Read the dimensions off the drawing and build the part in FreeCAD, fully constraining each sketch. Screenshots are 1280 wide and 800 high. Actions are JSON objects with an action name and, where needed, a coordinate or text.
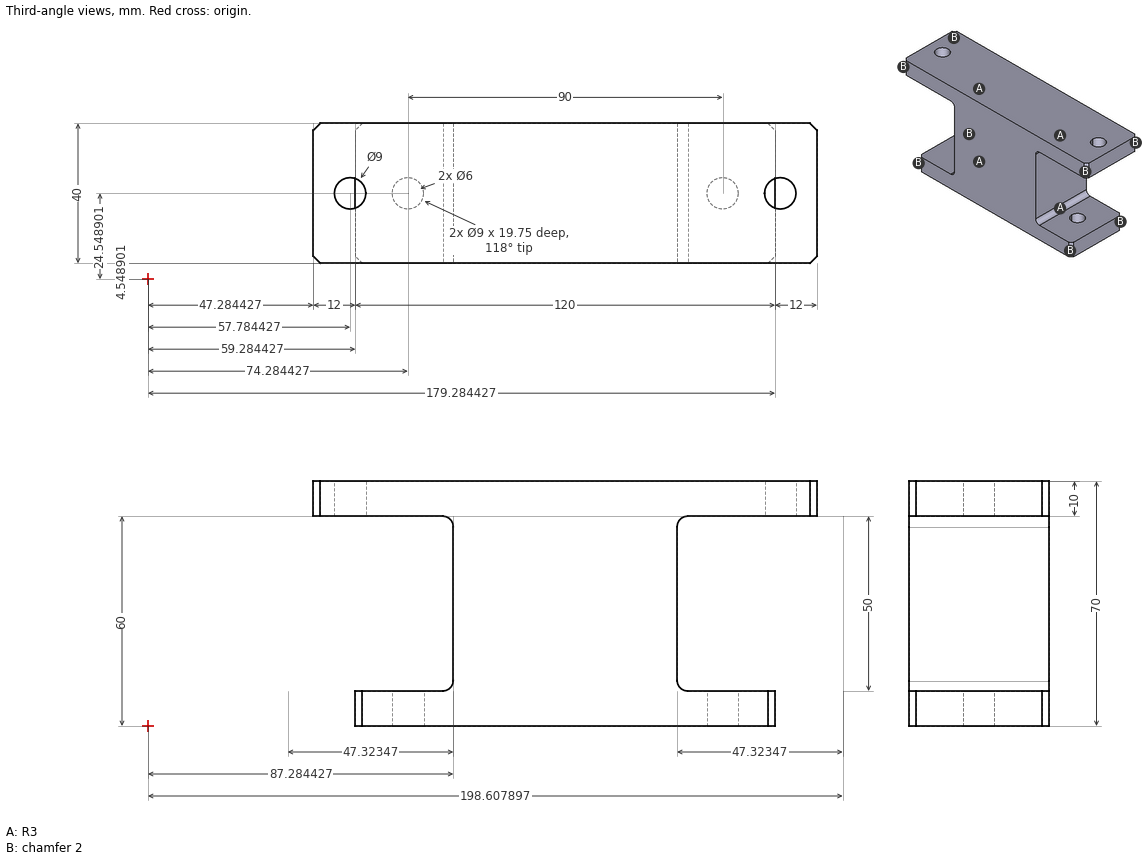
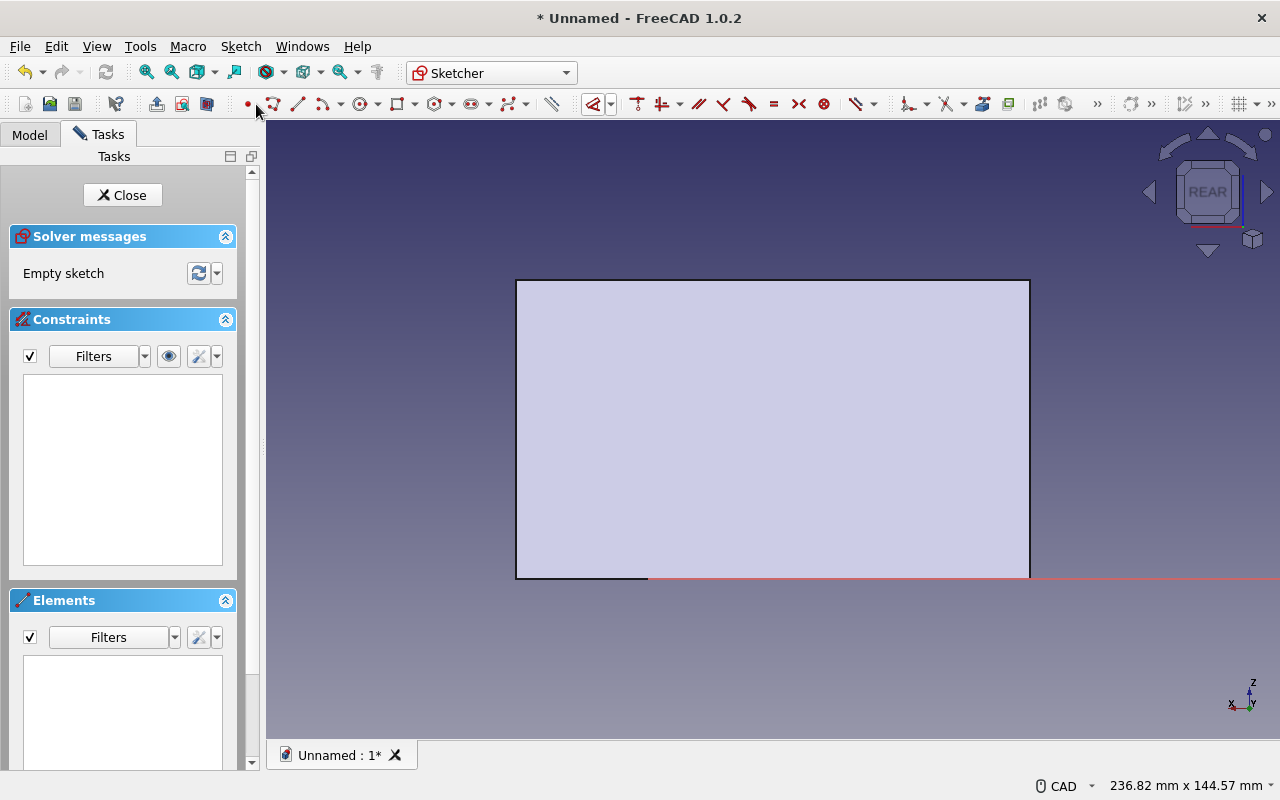
{"action": "scroll", "coordinate": [391, 386], "scroll_direction": "down", "scroll_amount": 2}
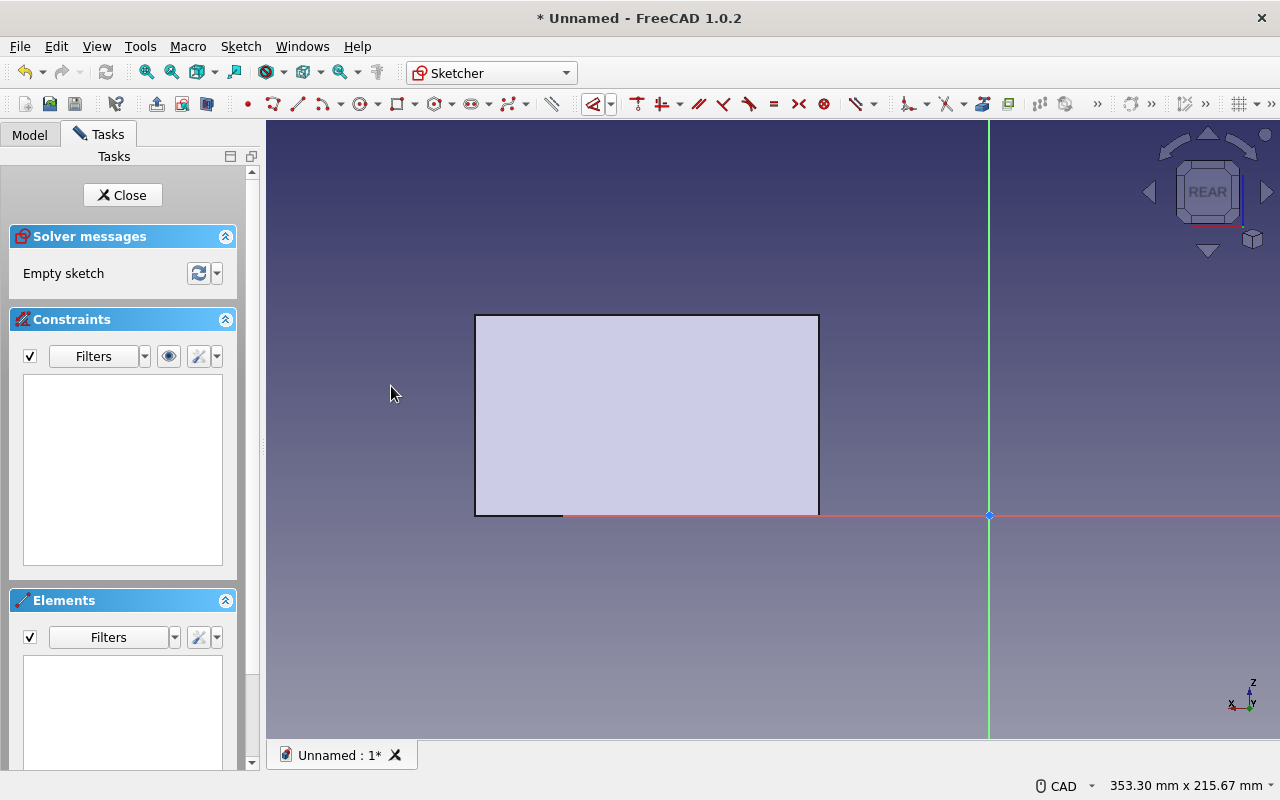
{"action": "left_click", "coordinate": [396, 104]}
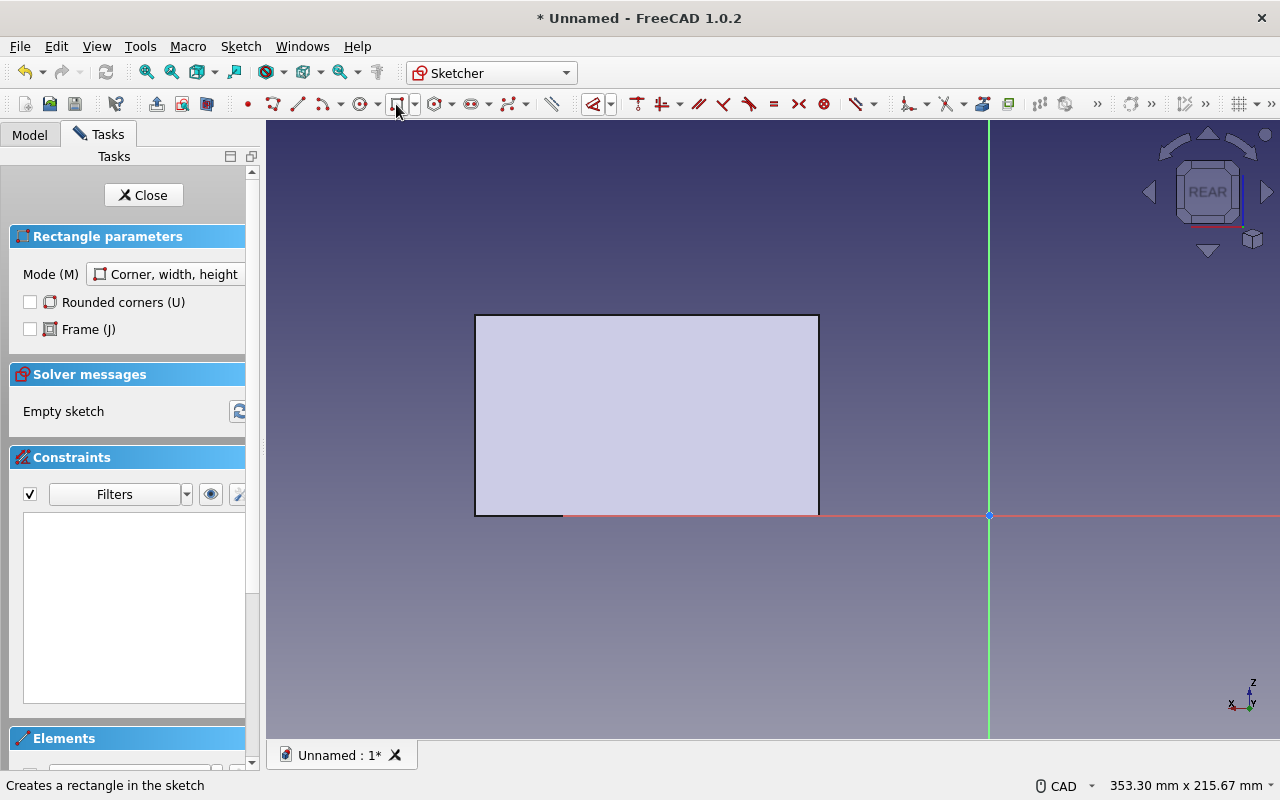
{"action": "left_click", "coordinate": [419, 344]}
{"action": "left_click", "coordinate": [555, 487]}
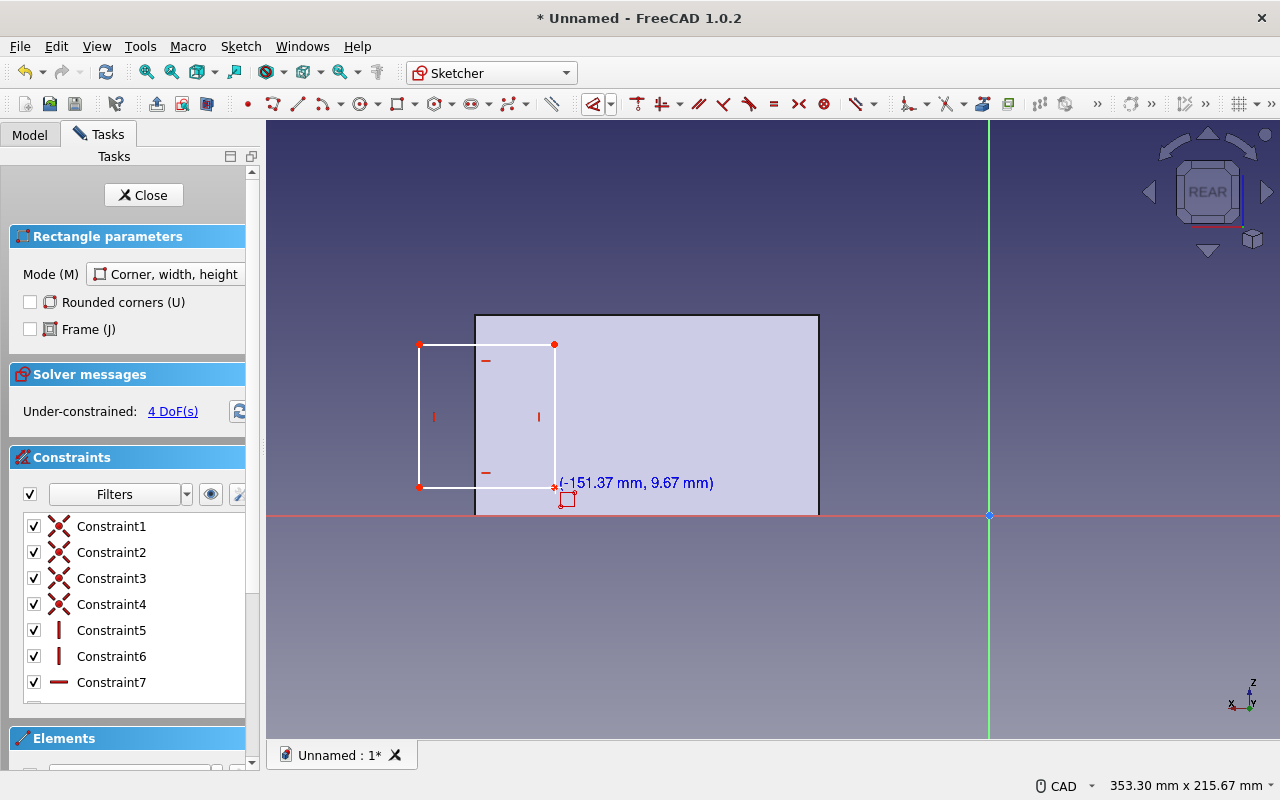
{"action": "left_click", "coordinate": [739, 344]}
{"action": "left_click", "coordinate": [875, 487]}
{"action": "key", "text": "Escape"}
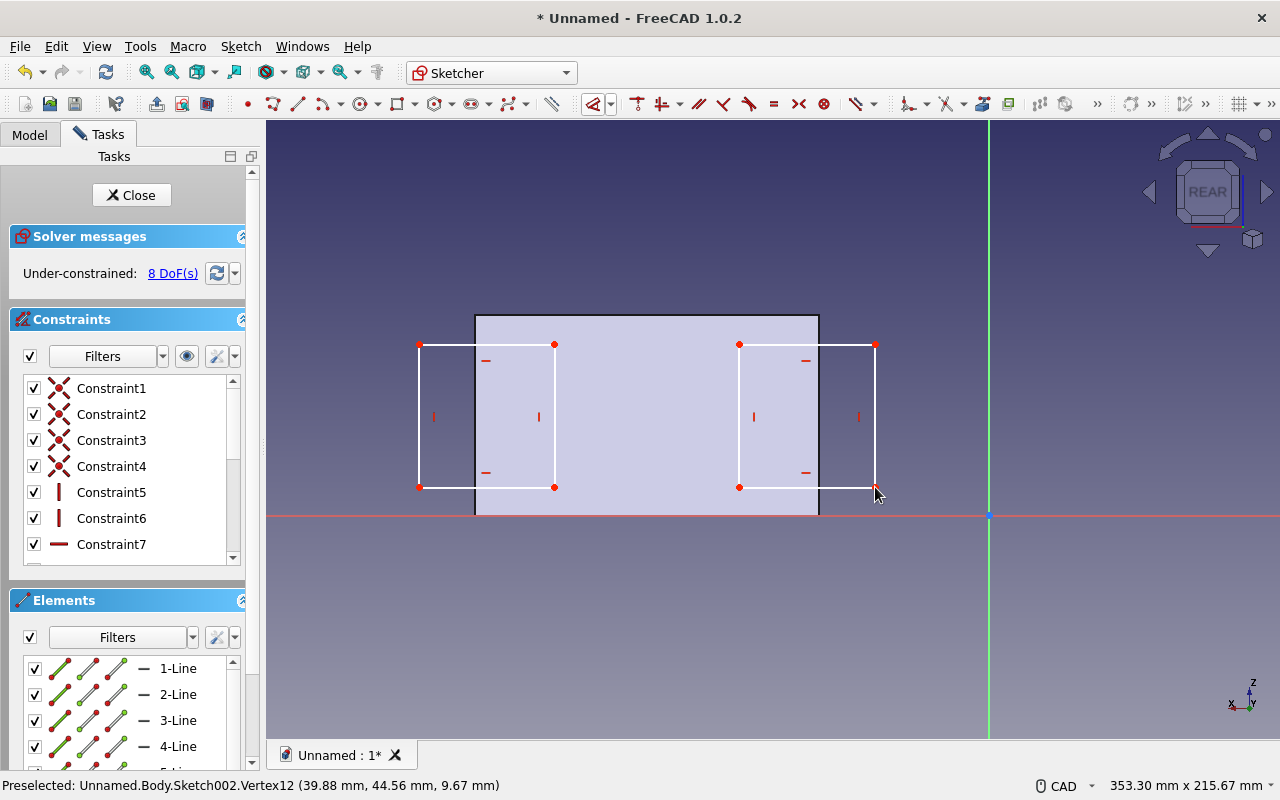
{"action": "left_click", "coordinate": [419, 388]}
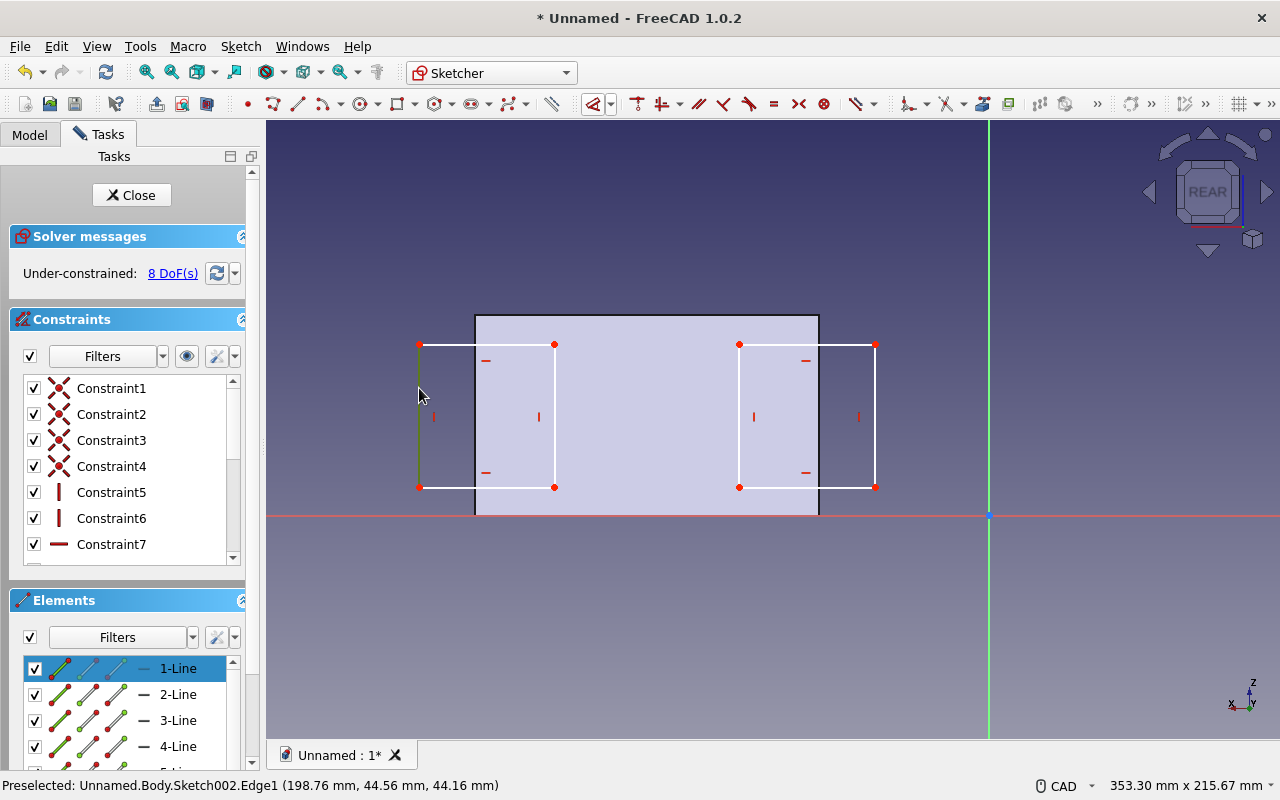
{"action": "left_click", "coordinate": [610, 104]}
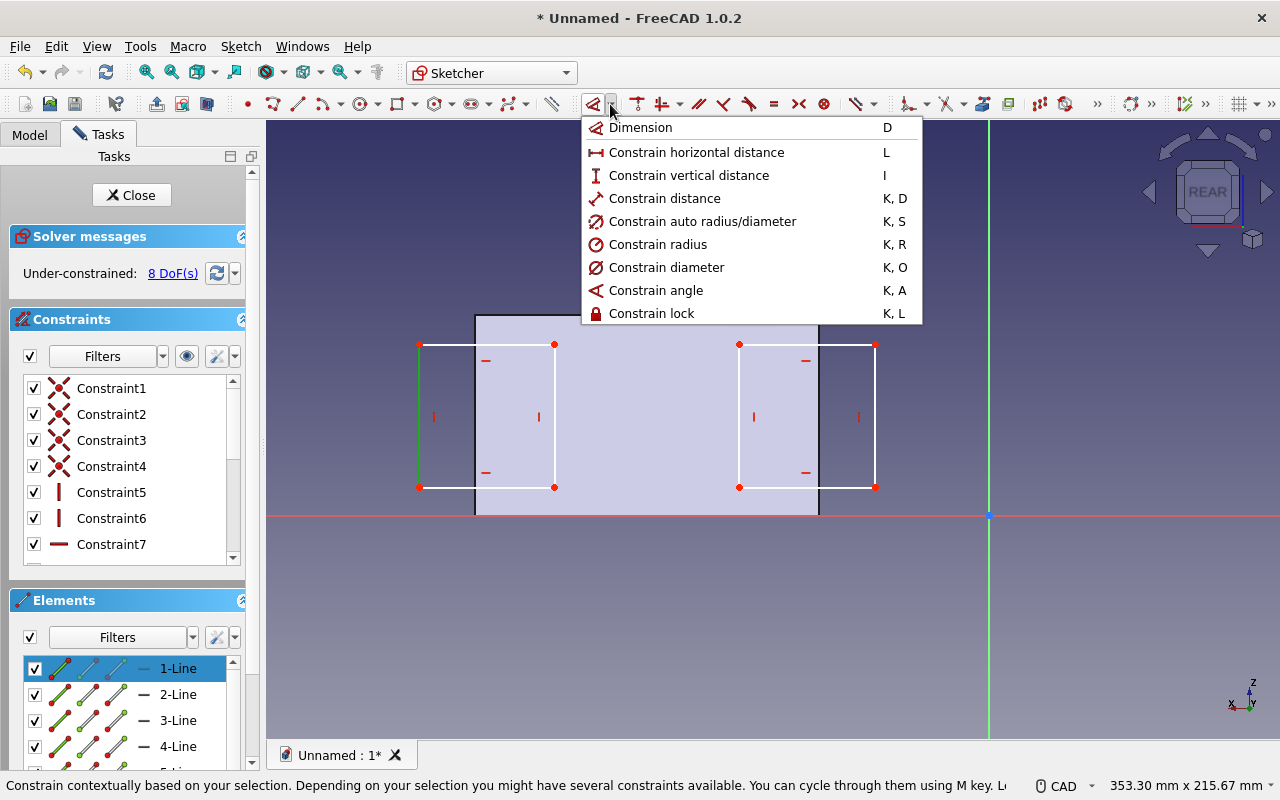
{"action": "left_click", "coordinate": [752, 176]}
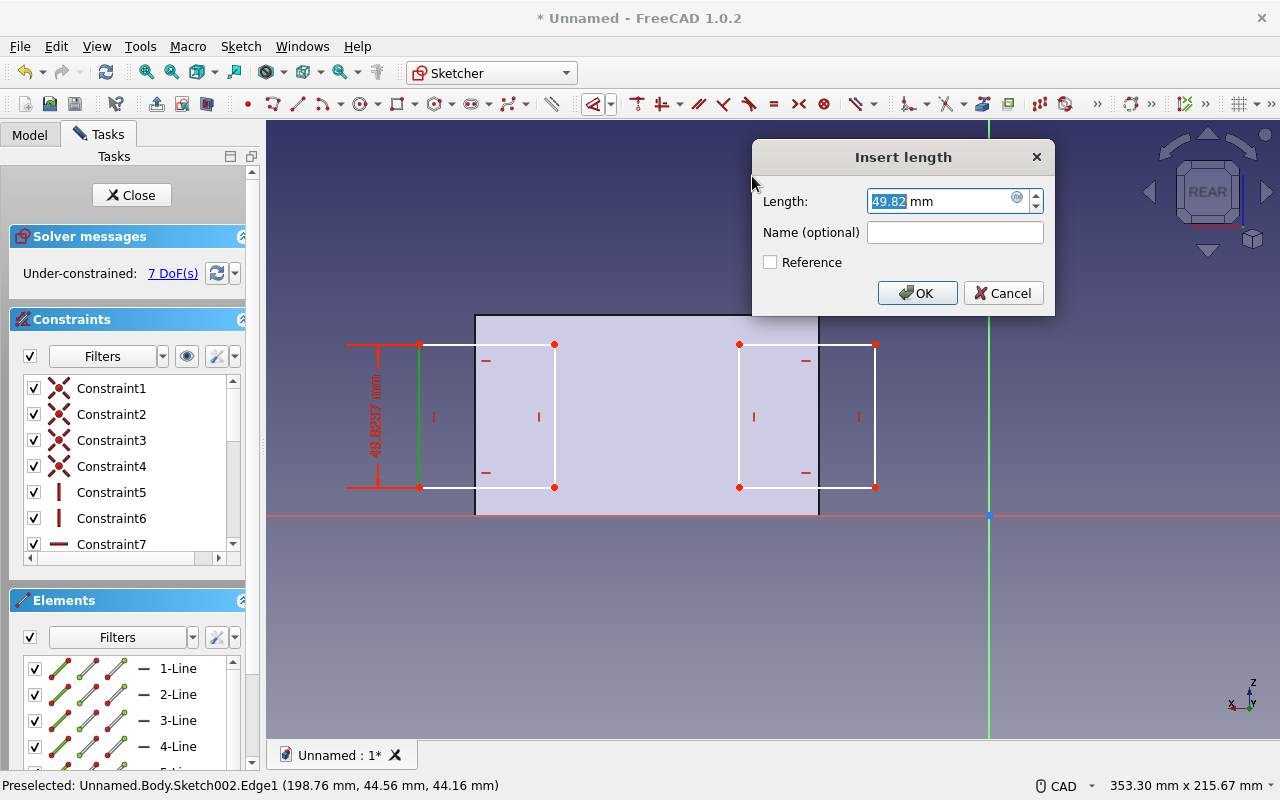
{"action": "type", "text": "50"}
{"action": "key", "text": "Return"}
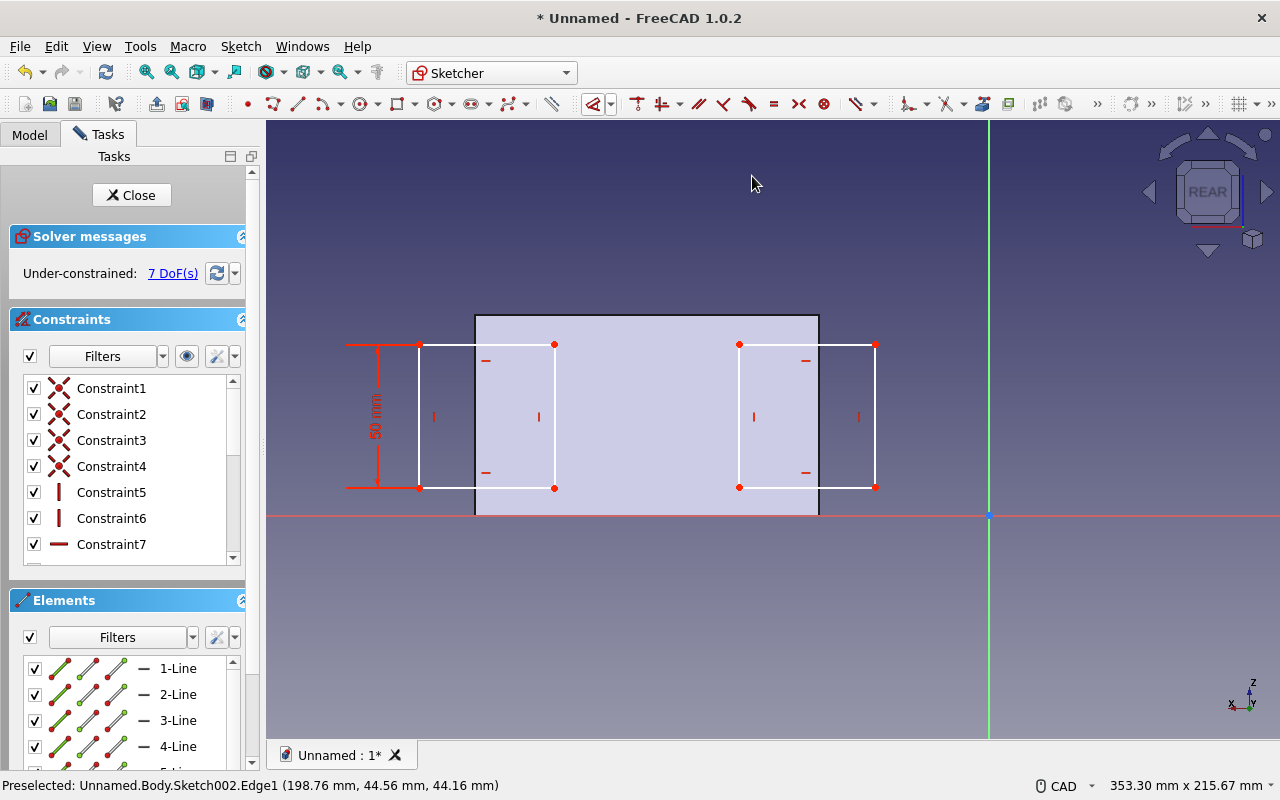
{"action": "left_click", "coordinate": [739, 388]}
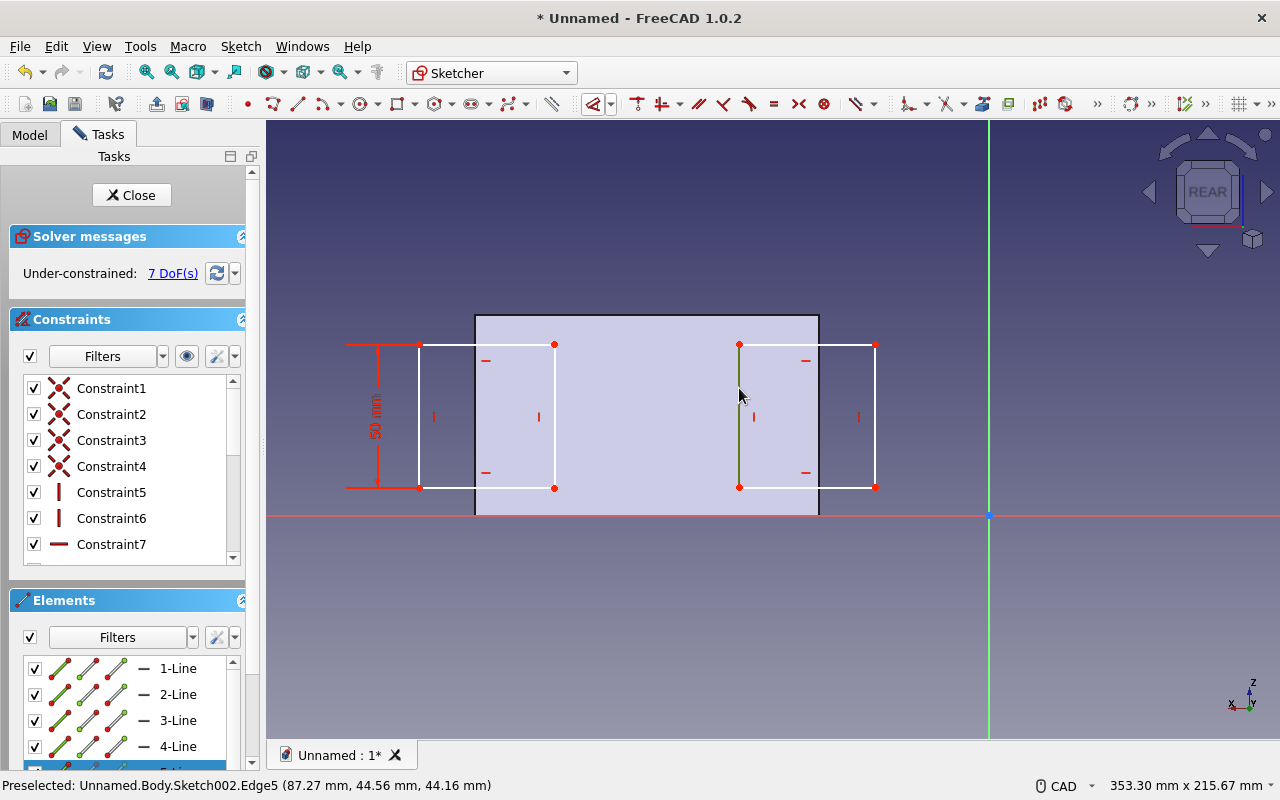
{"action": "key", "text": "i"}